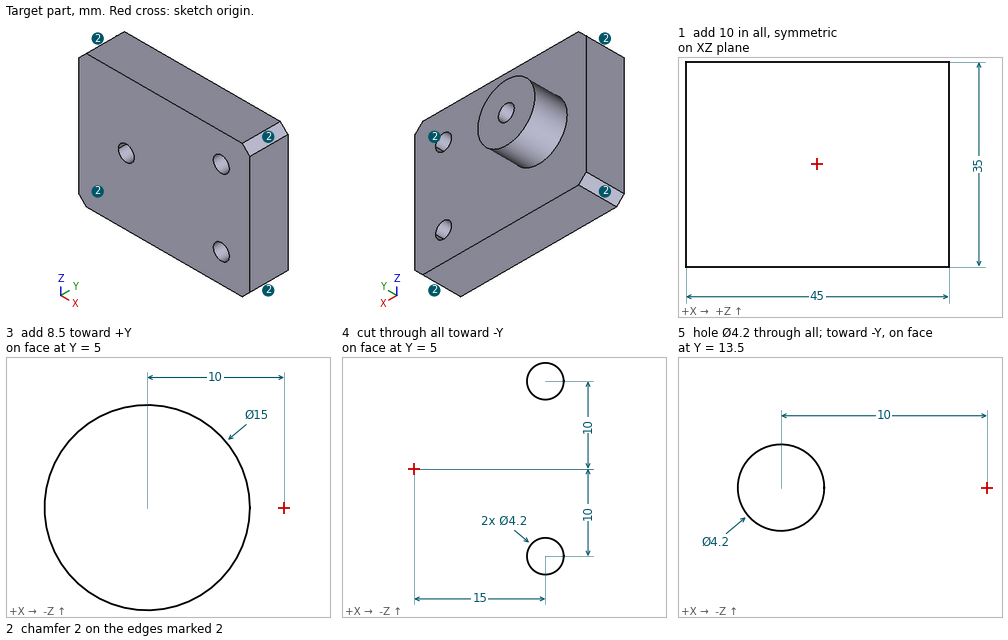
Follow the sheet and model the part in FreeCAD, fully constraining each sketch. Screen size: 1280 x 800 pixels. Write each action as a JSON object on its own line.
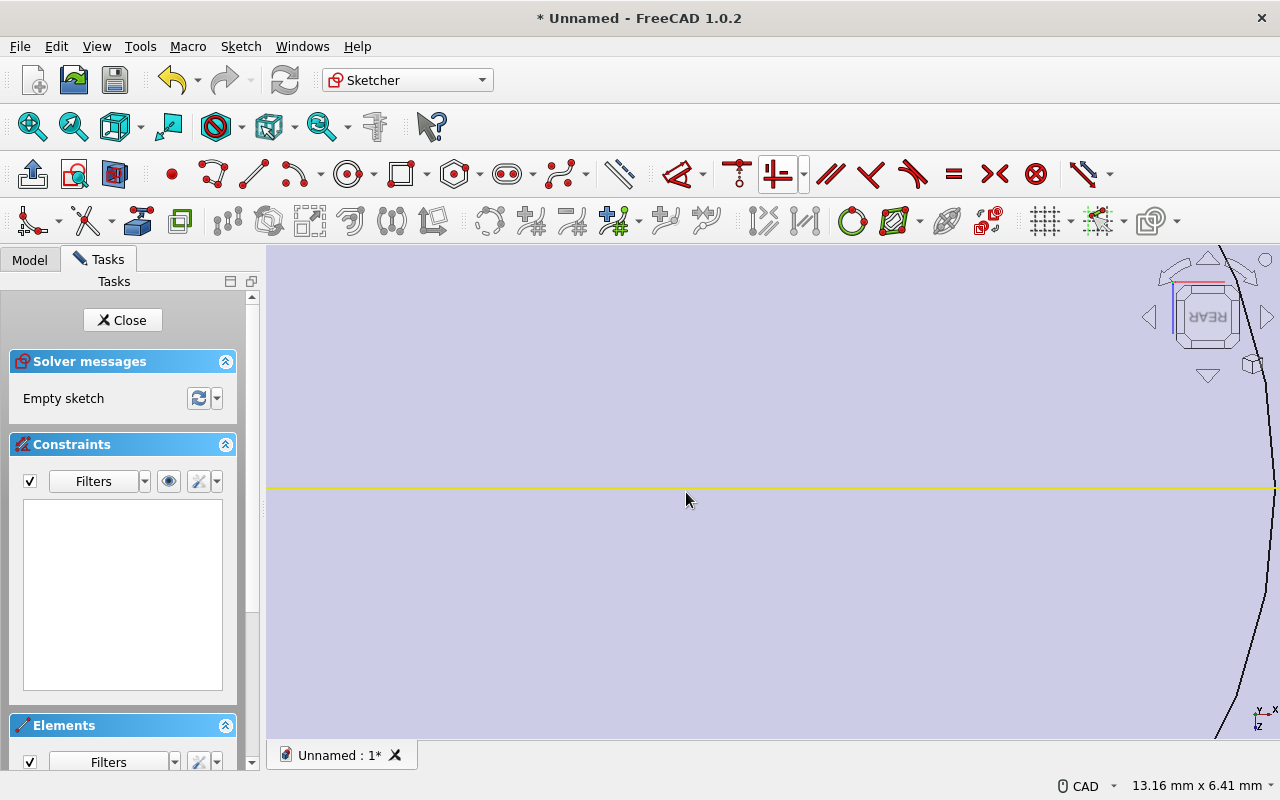
{"action": "key", "text": "g c"}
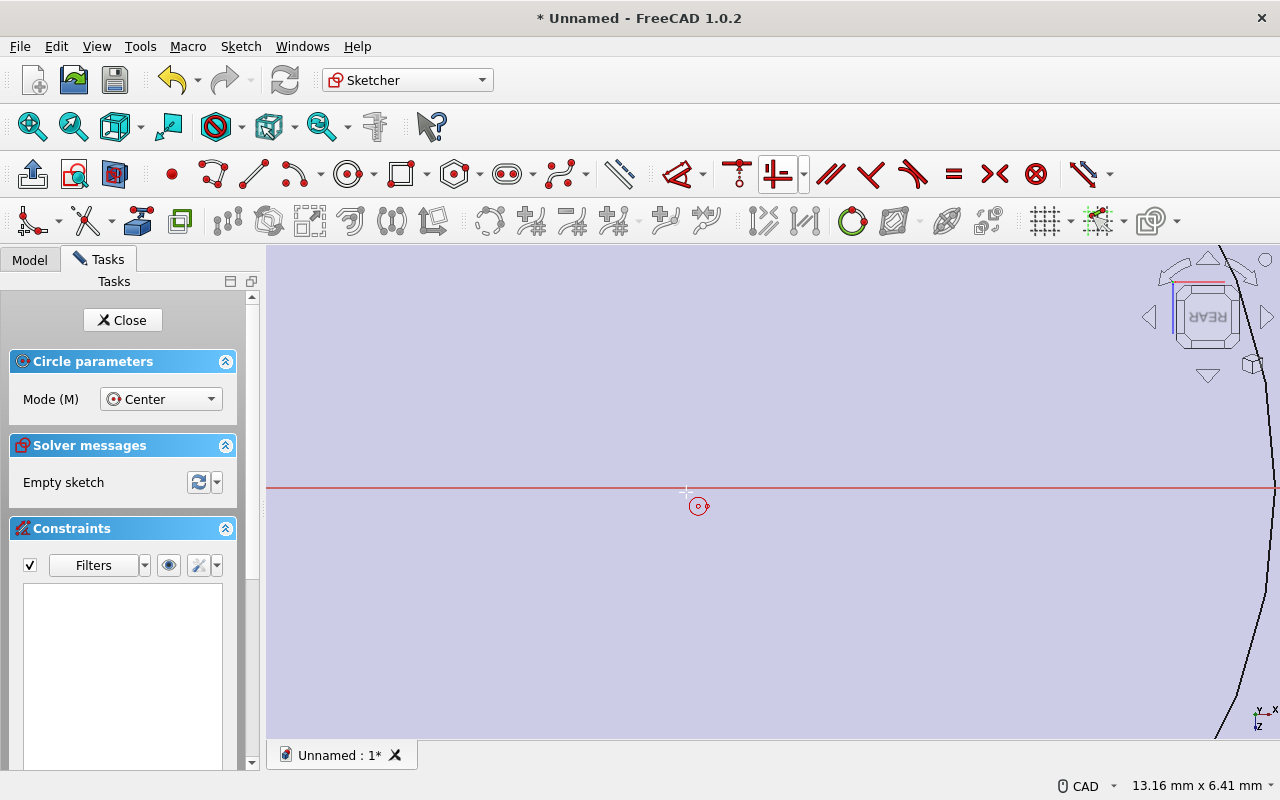
{"action": "left_click", "coordinate": [698, 488]}
{"action": "mouse_move", "coordinate": [812, 374]}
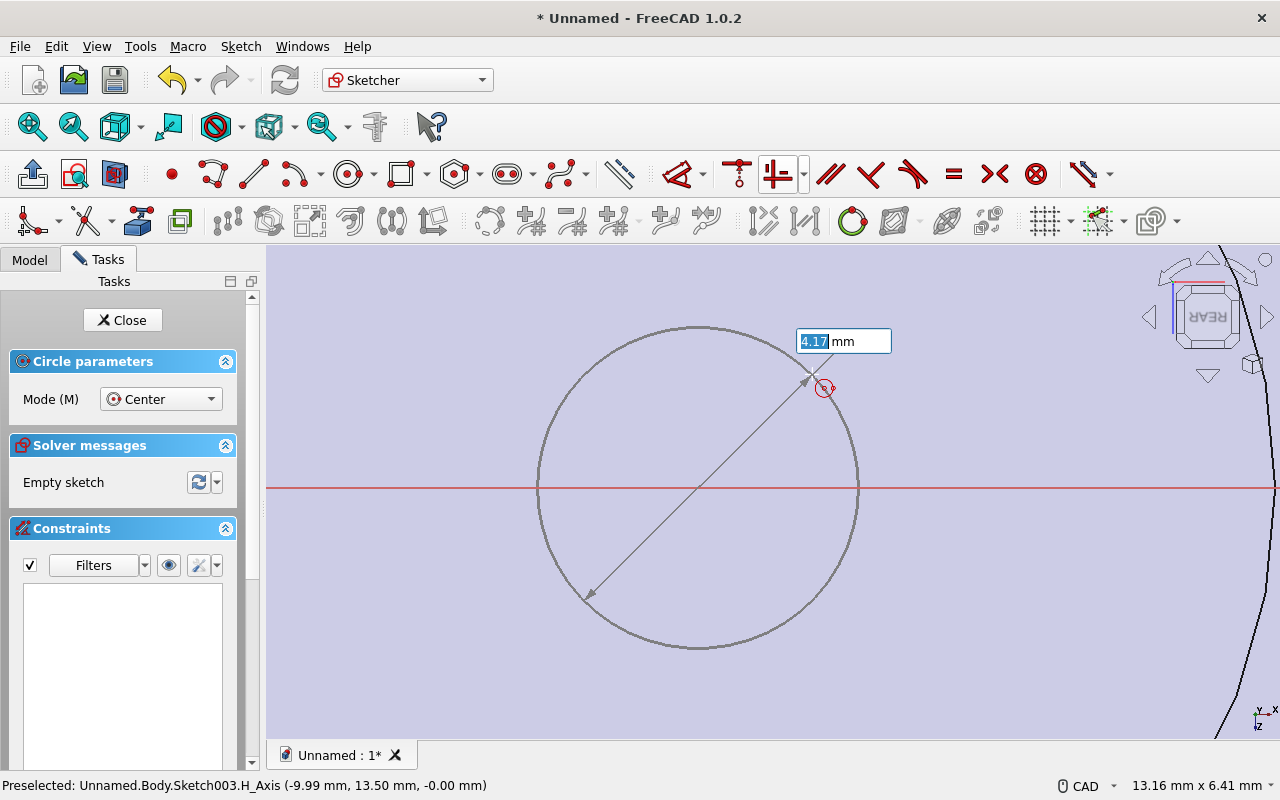
{"action": "type", "text": "4.2"}
{"action": "key", "text": "Return"}
{"action": "key", "text": "Escape"}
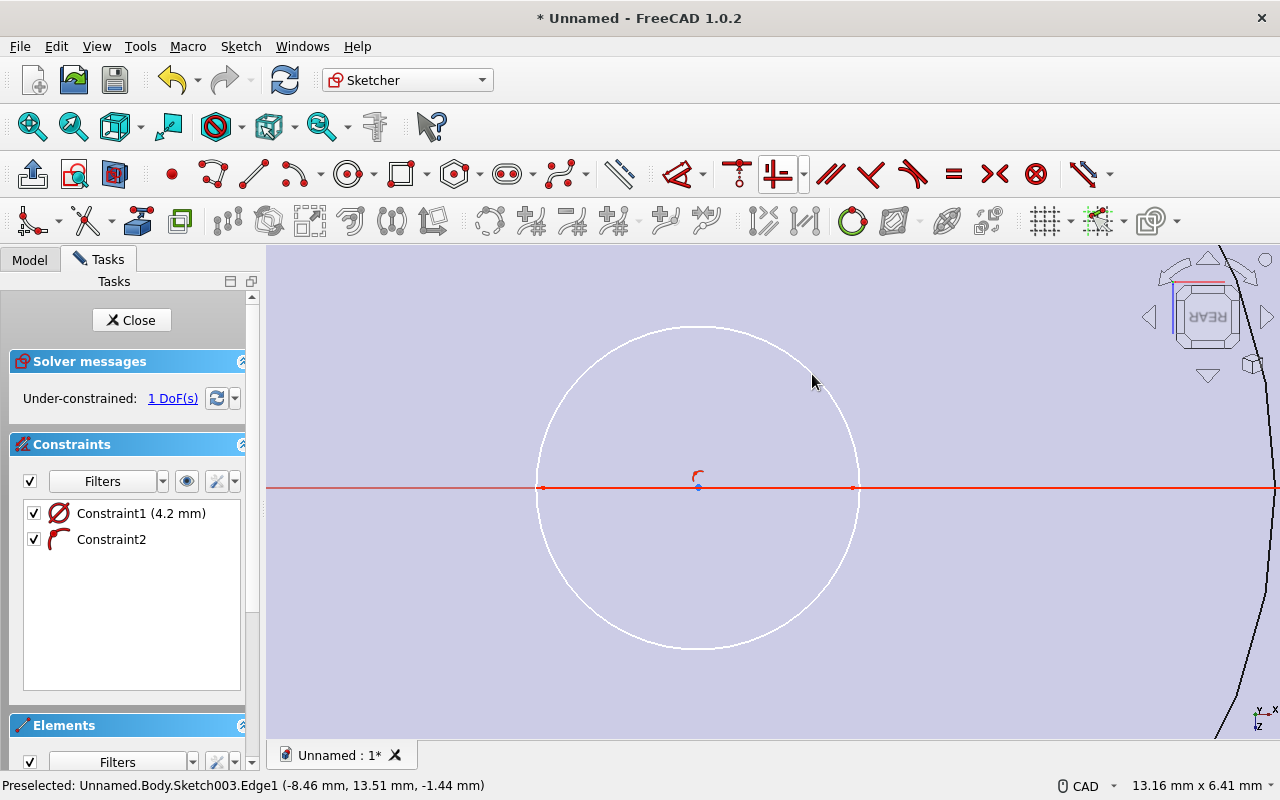
{"action": "left_click", "coordinate": [676, 174]}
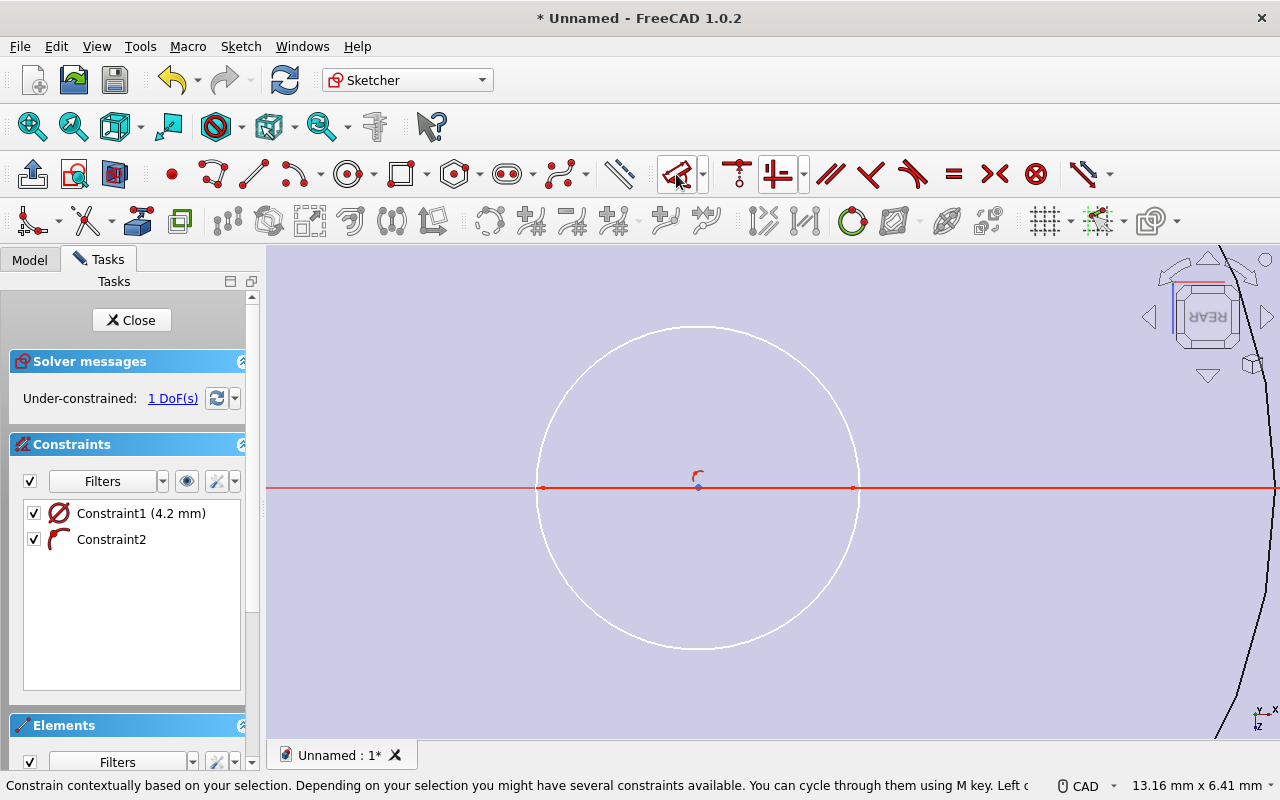
{"action": "left_click", "coordinate": [698, 488]}
{"action": "left_click", "coordinate": [907, 522]}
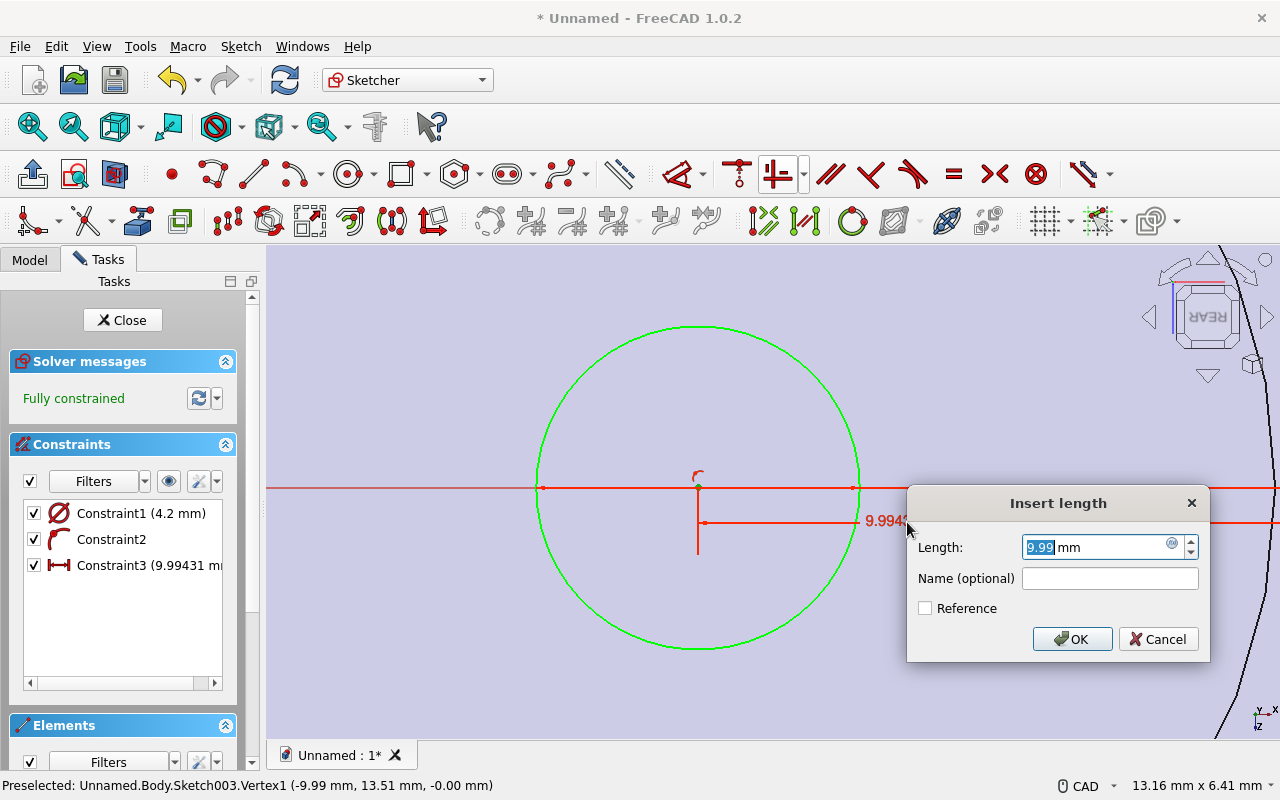
{"action": "type", "text": "10"}
{"action": "key", "text": "Return"}
{"action": "key", "text": "Escape"}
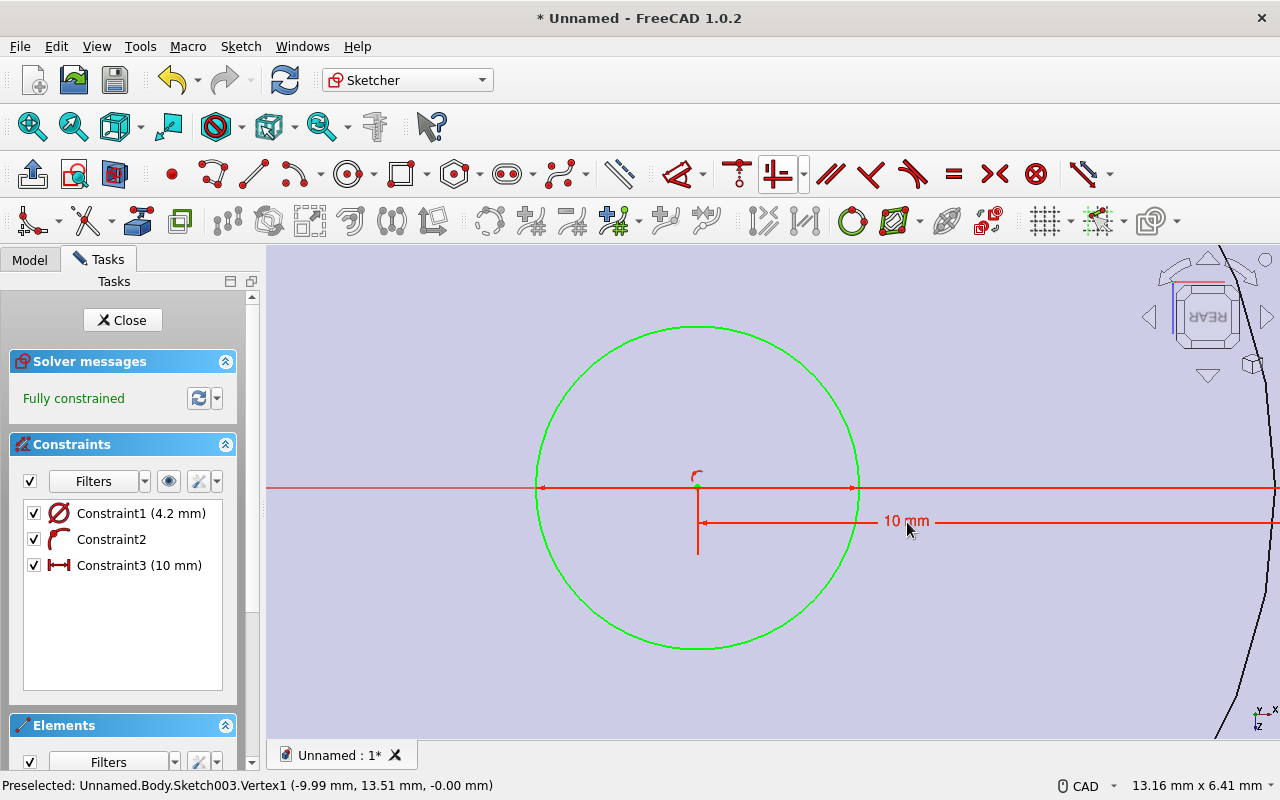
{"action": "left_click", "coordinate": [123, 320]}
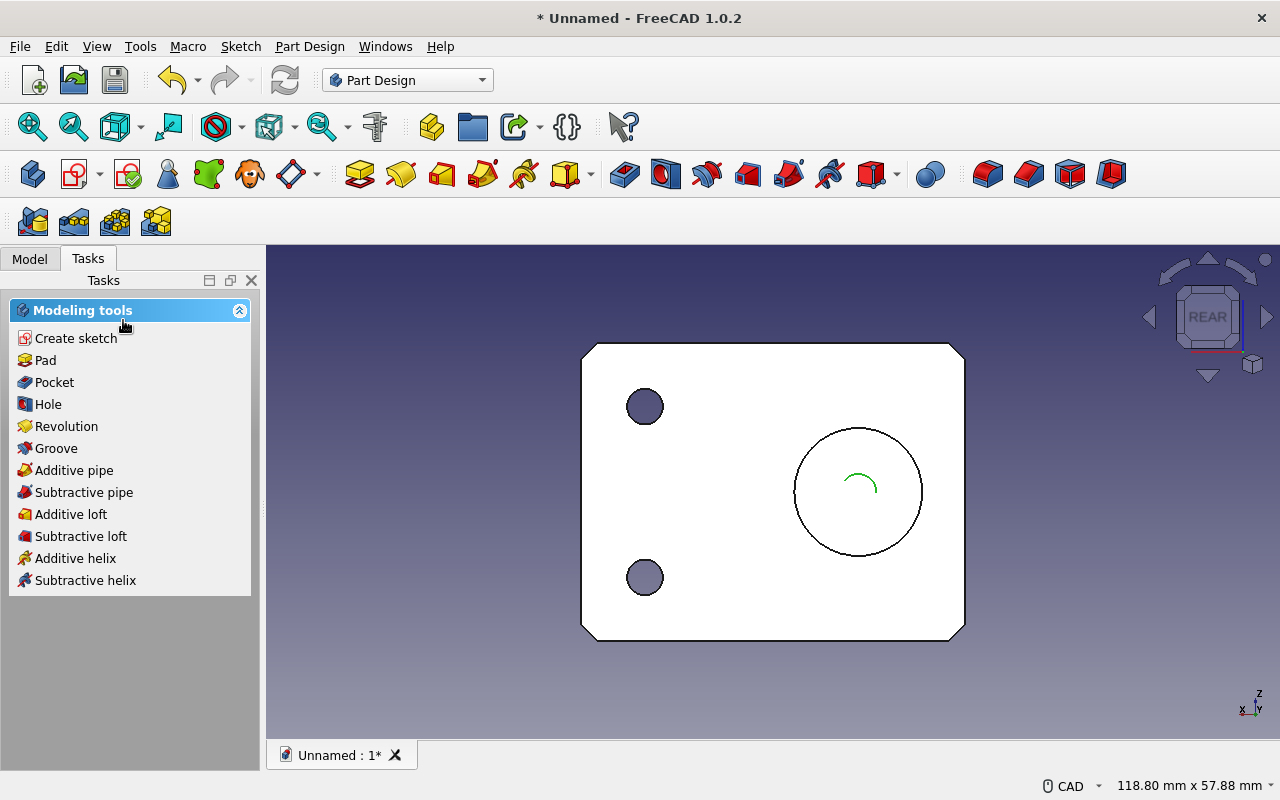
{"action": "left_click", "coordinate": [666, 174]}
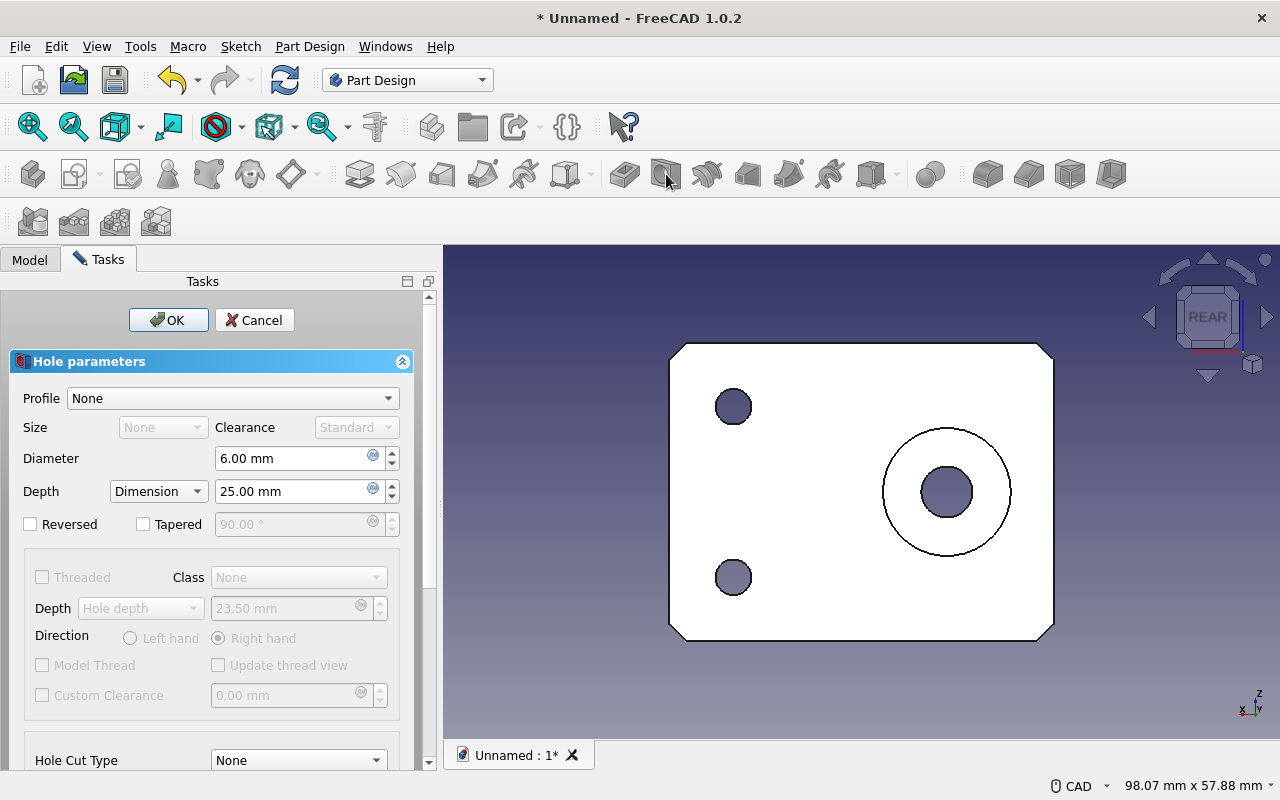
{"action": "triple_click", "coordinate": [300, 458]}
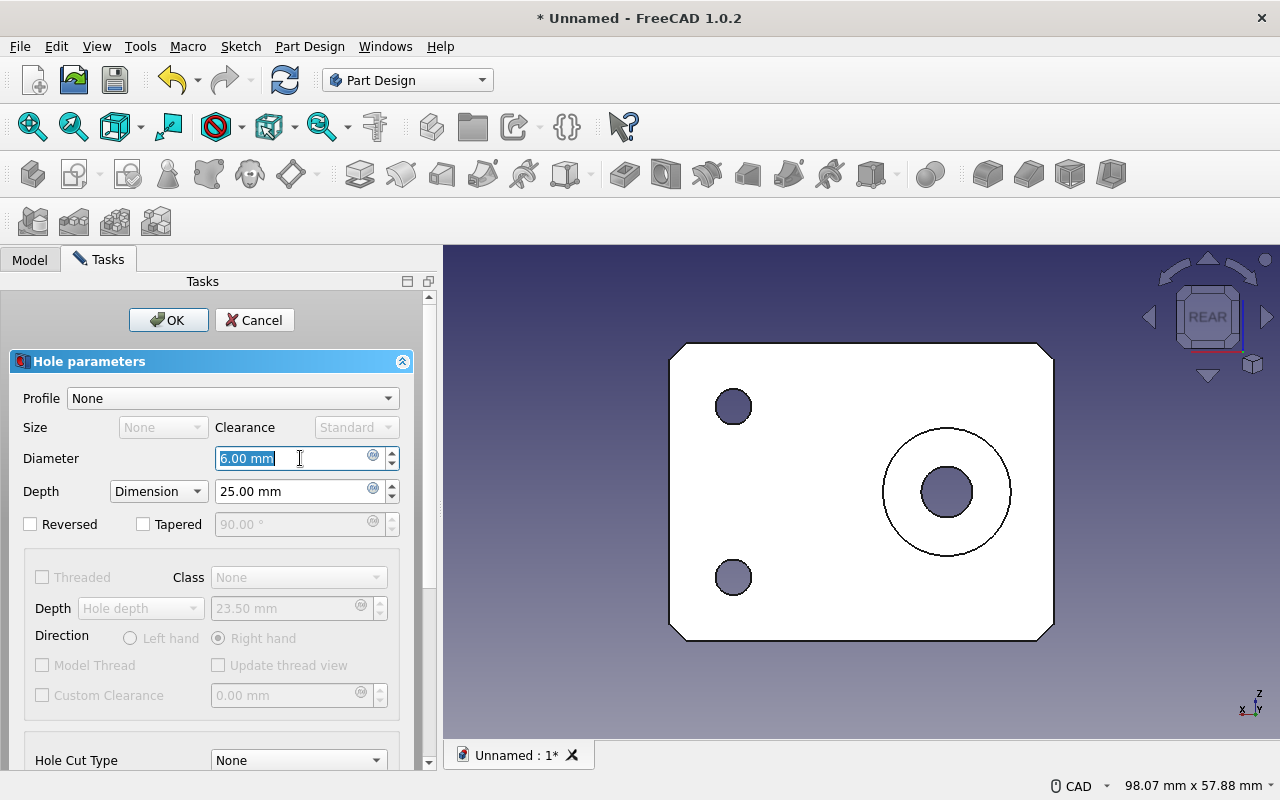
{"action": "type", "text": "4.2"}
{"action": "key", "text": "Tab"}